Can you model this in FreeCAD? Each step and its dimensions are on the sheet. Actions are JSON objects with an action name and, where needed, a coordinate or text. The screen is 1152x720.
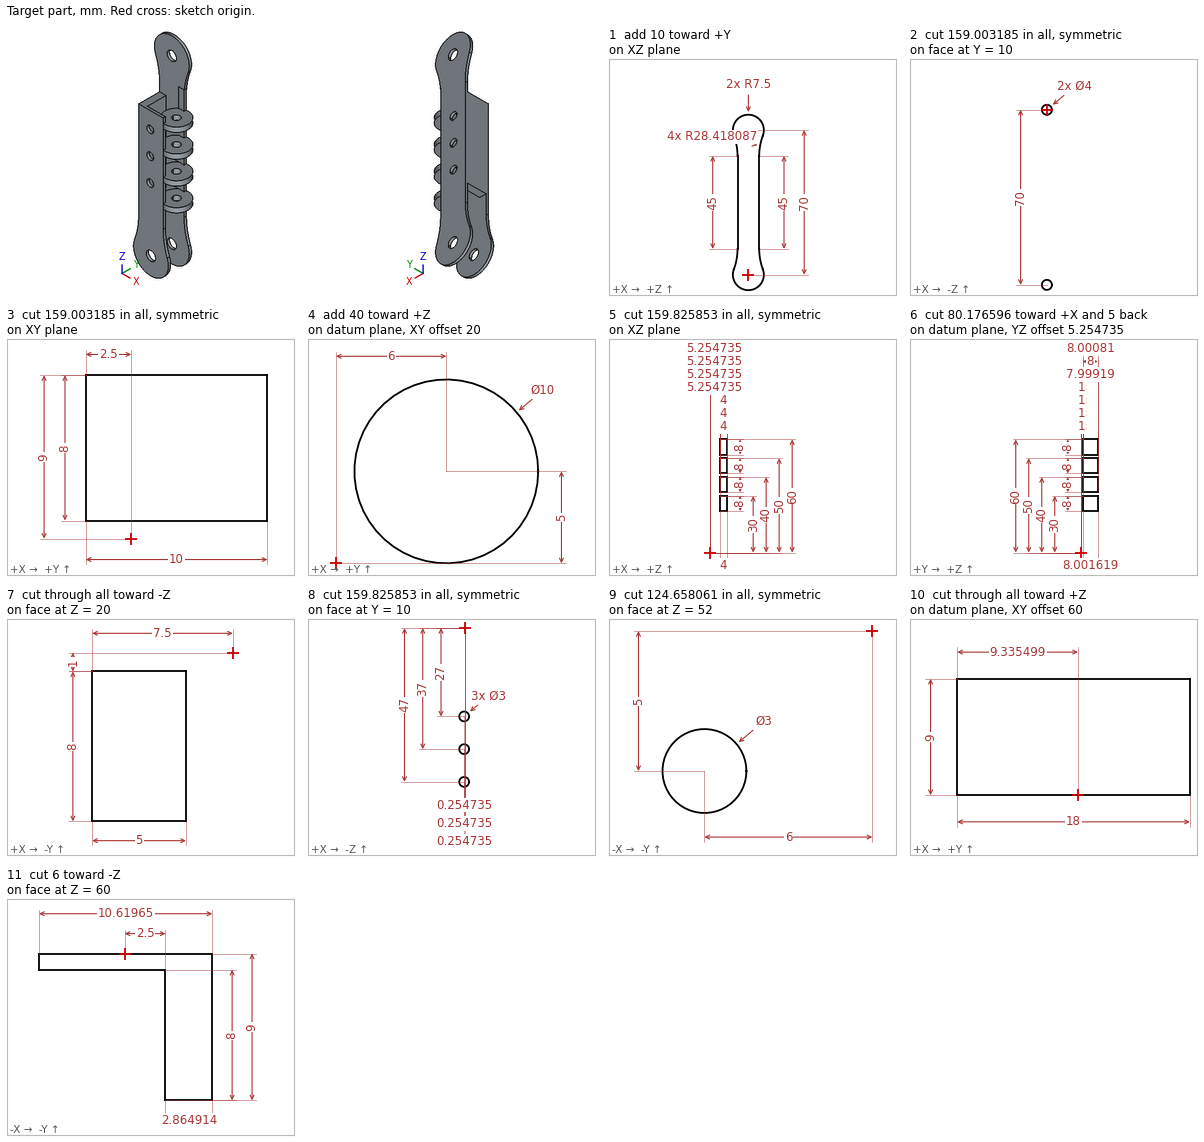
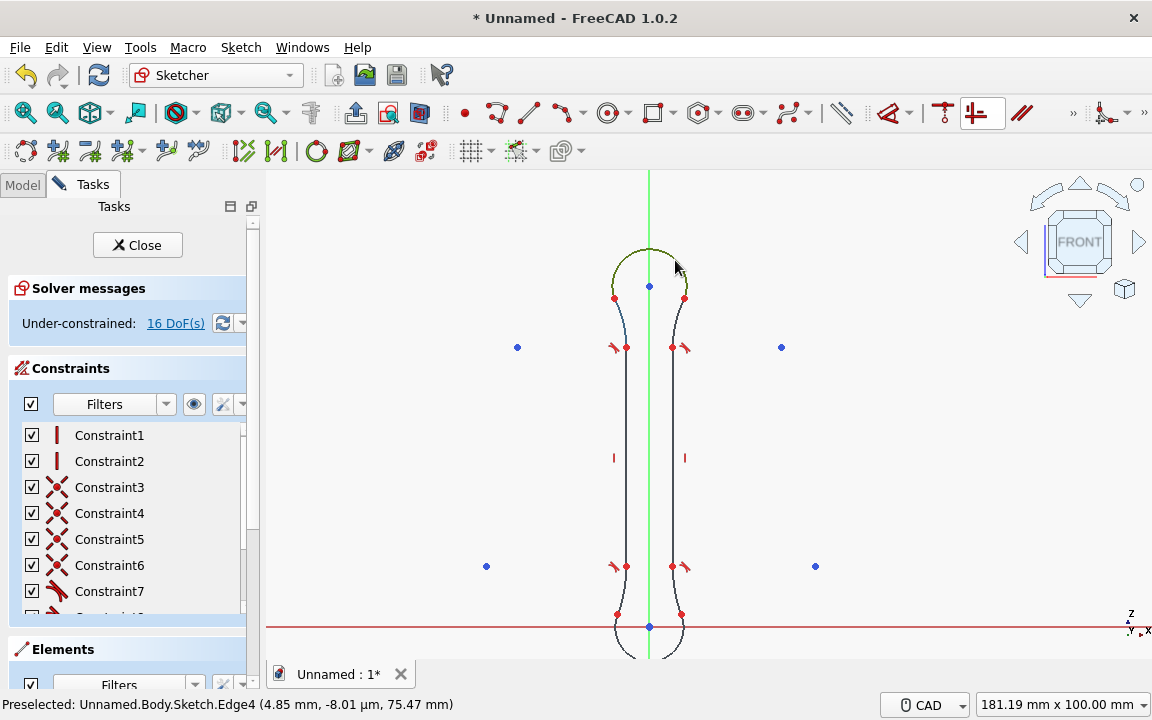
{"action": "key", "text": "t"}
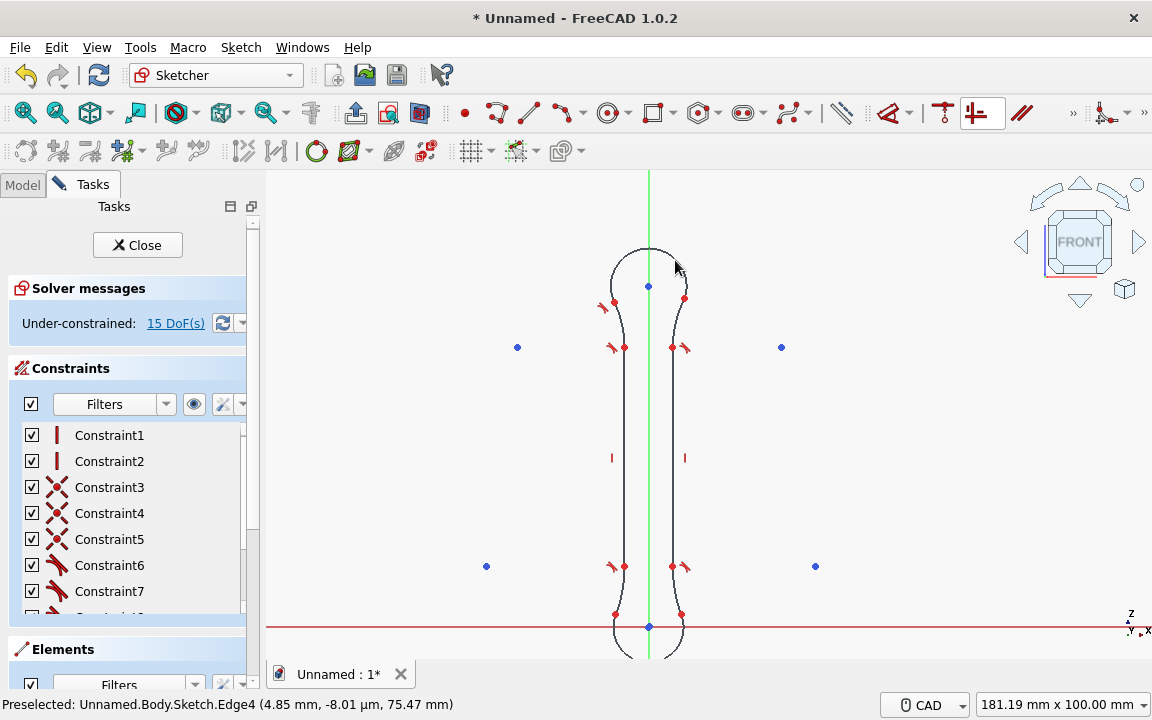
{"action": "left_click", "coordinate": [674, 258]}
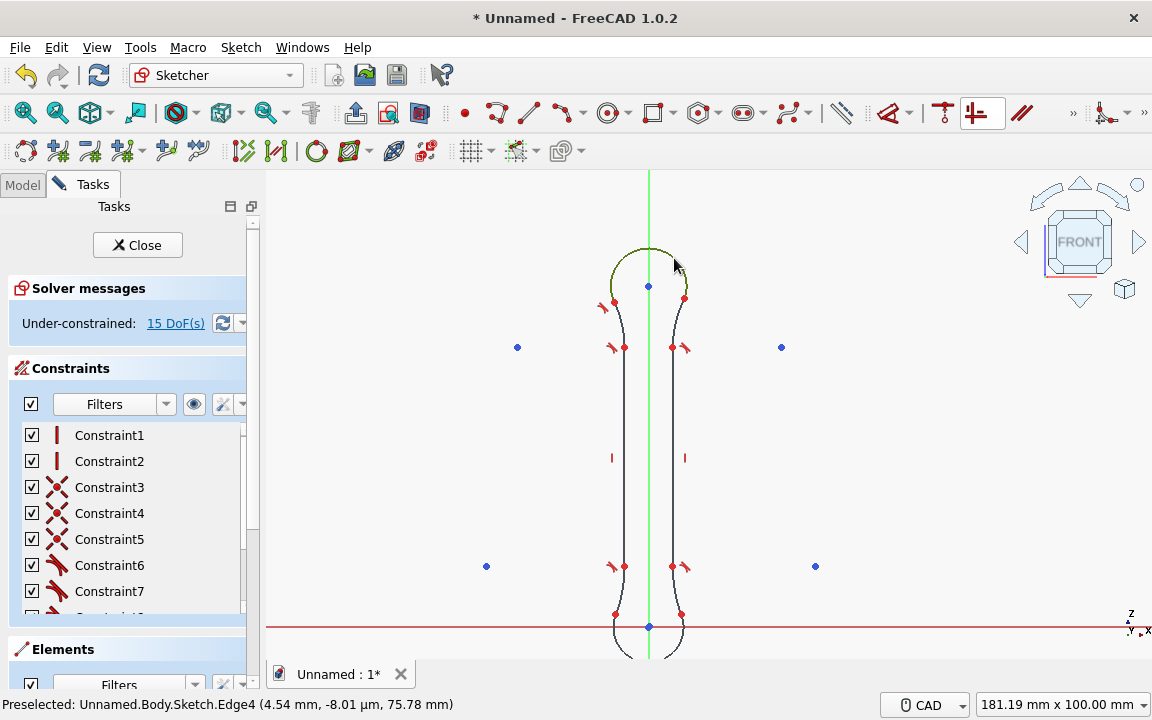
{"action": "left_click", "coordinate": [679, 313]}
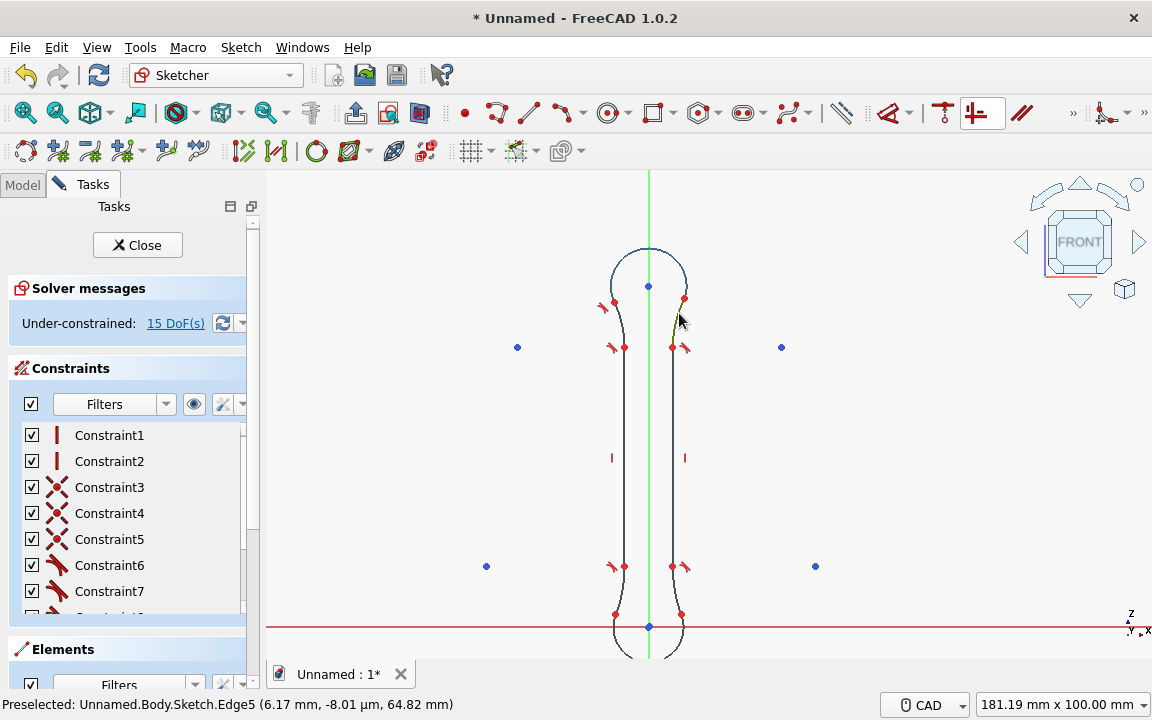
{"action": "key", "text": "t"}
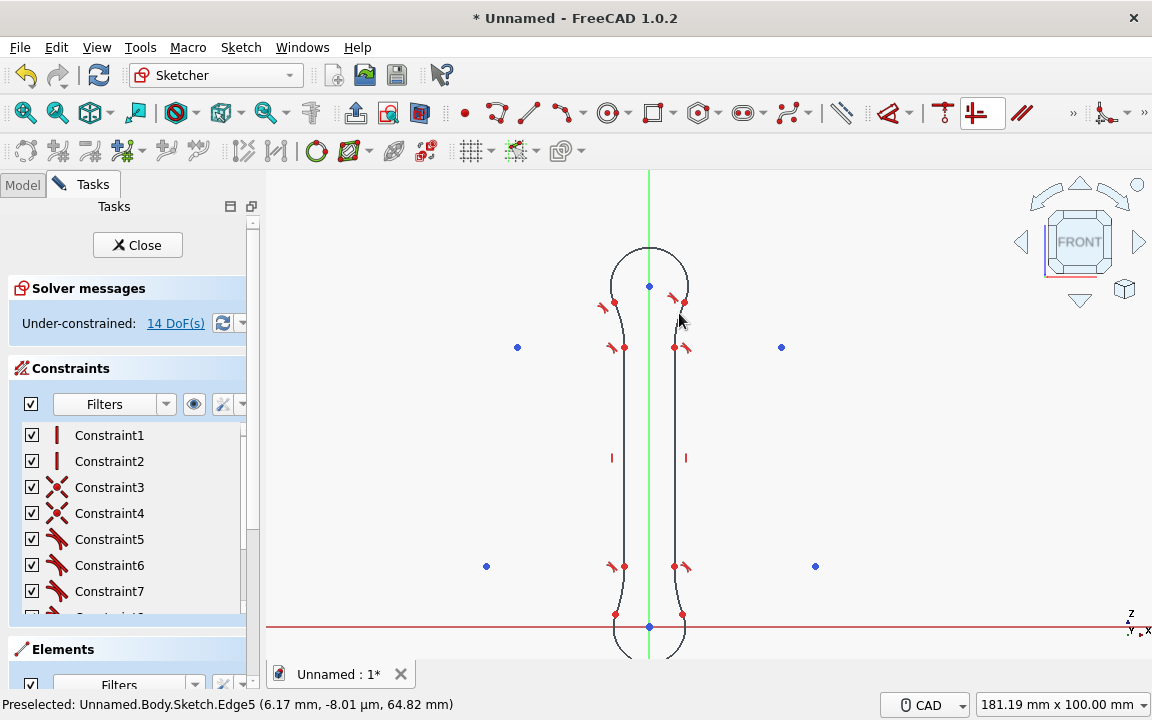
{"action": "left_click", "coordinate": [675, 582]}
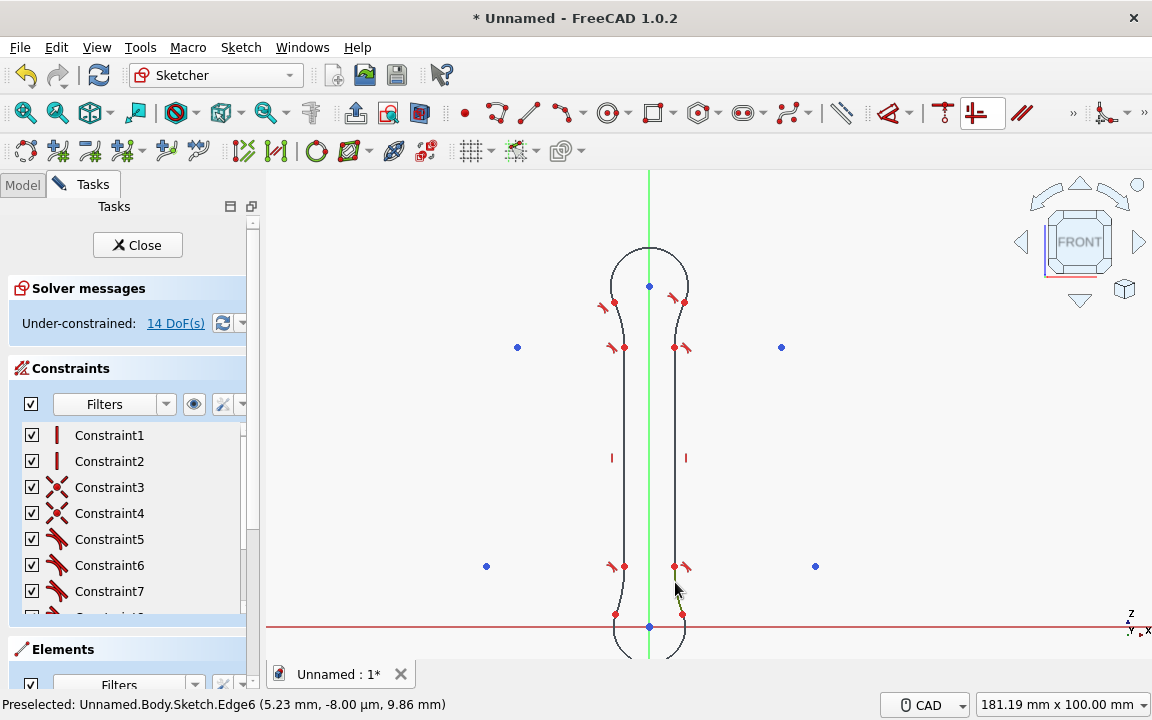
{"action": "scroll", "coordinate": [622, 331], "scroll_direction": "down", "scroll_amount": 2}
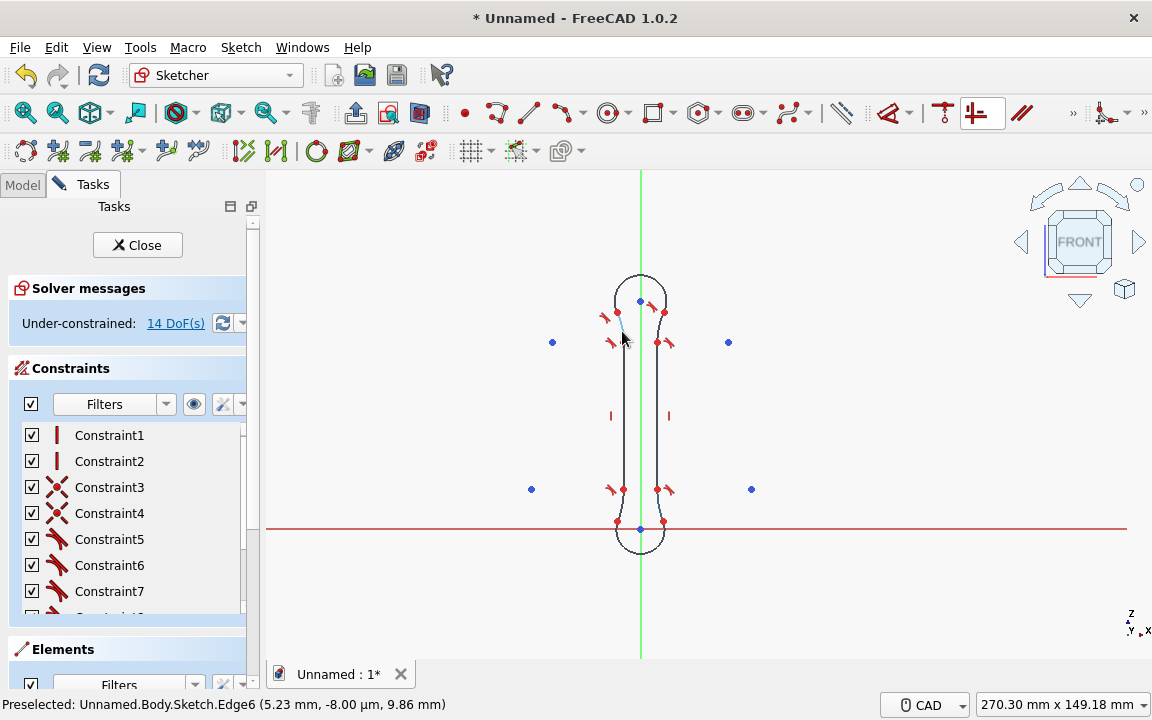
{"action": "left_click", "coordinate": [624, 547]}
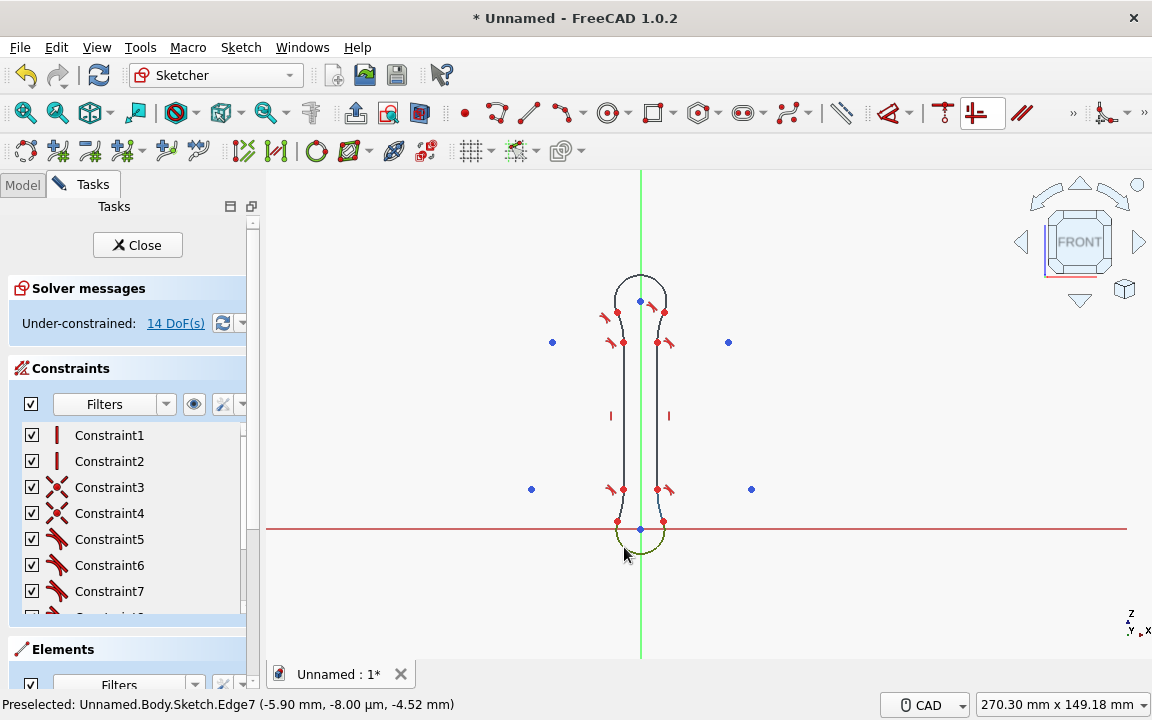
{"action": "key", "text": "t"}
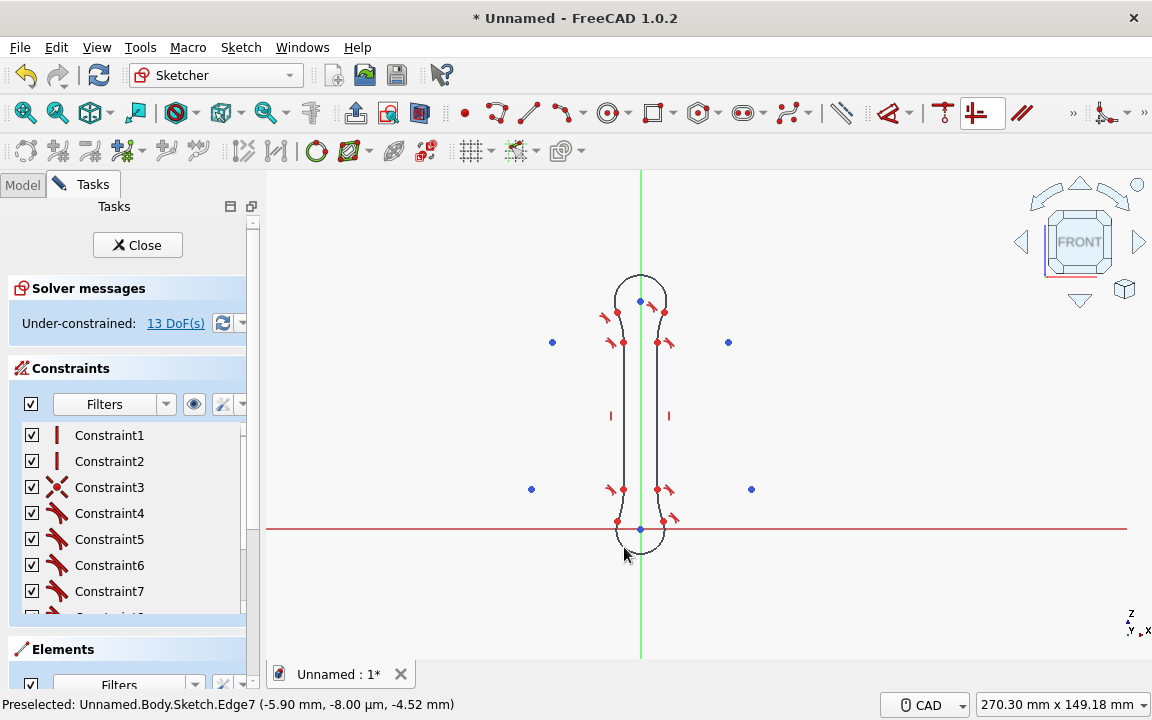
{"action": "left_click", "coordinate": [624, 547]}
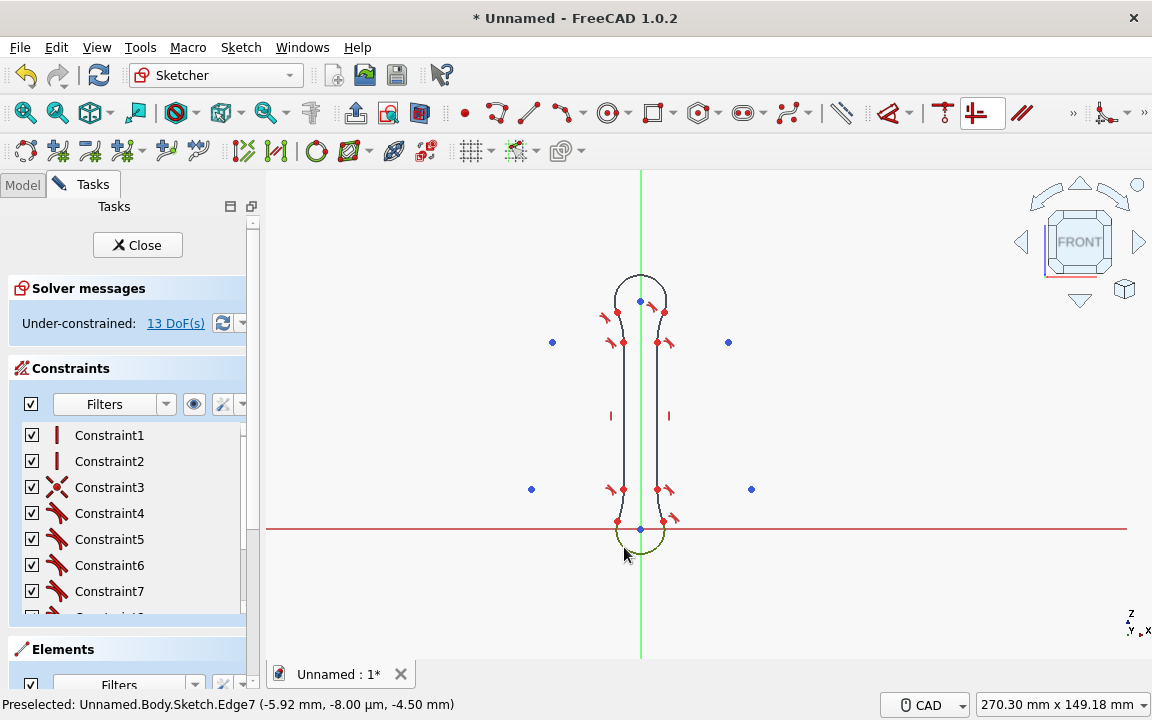
{"action": "scroll", "coordinate": [621, 512], "scroll_direction": "up", "scroll_amount": 2}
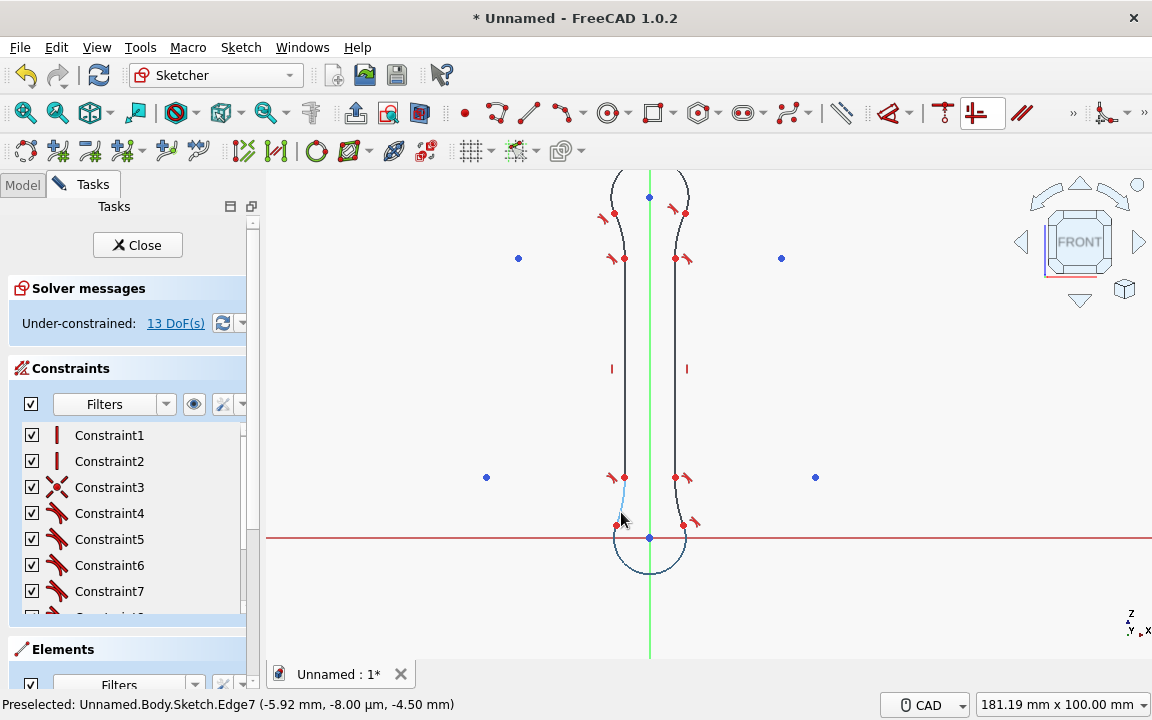
{"action": "left_click", "coordinate": [621, 511]}